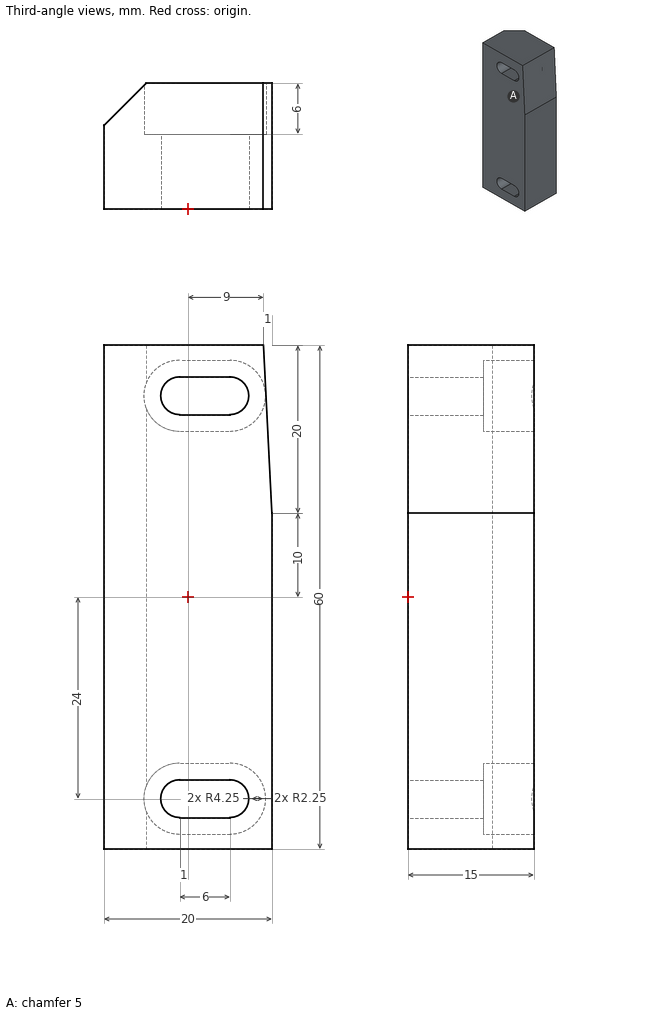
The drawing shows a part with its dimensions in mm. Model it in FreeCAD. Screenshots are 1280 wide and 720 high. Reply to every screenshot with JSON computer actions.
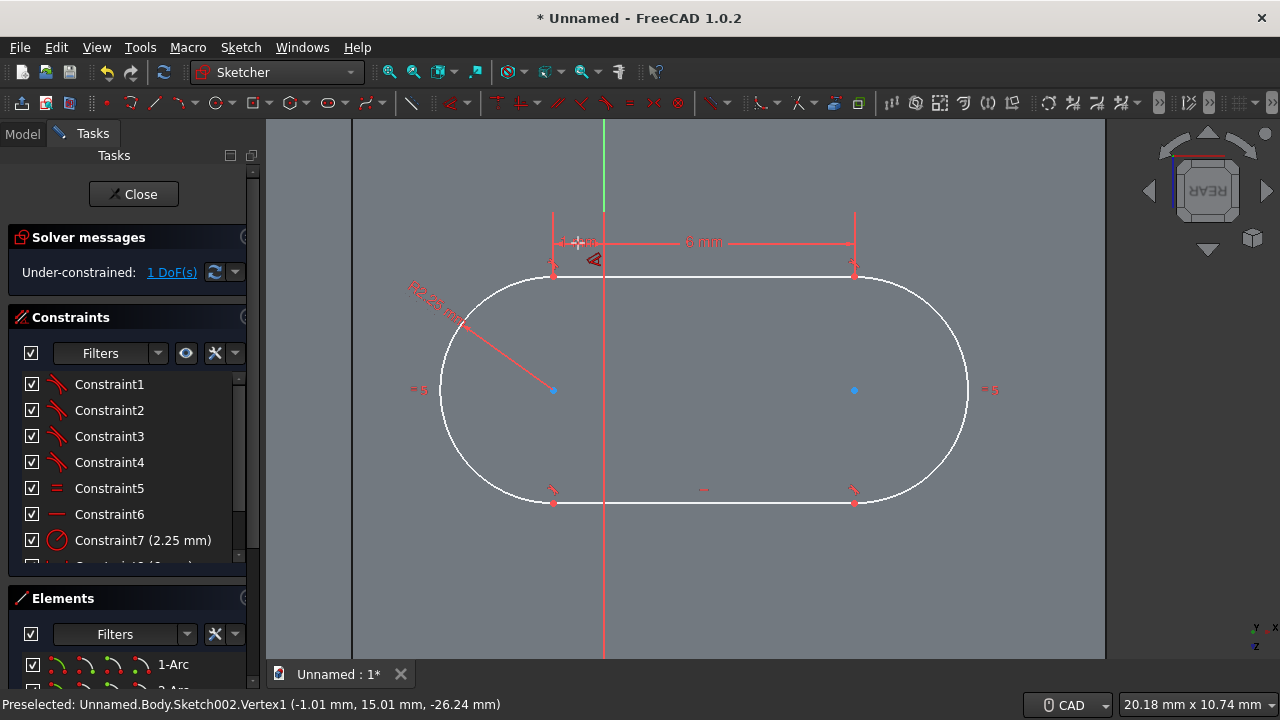
{"action": "left_click", "coordinate": [553, 390]}
{"action": "left_click", "coordinate": [519, 455]}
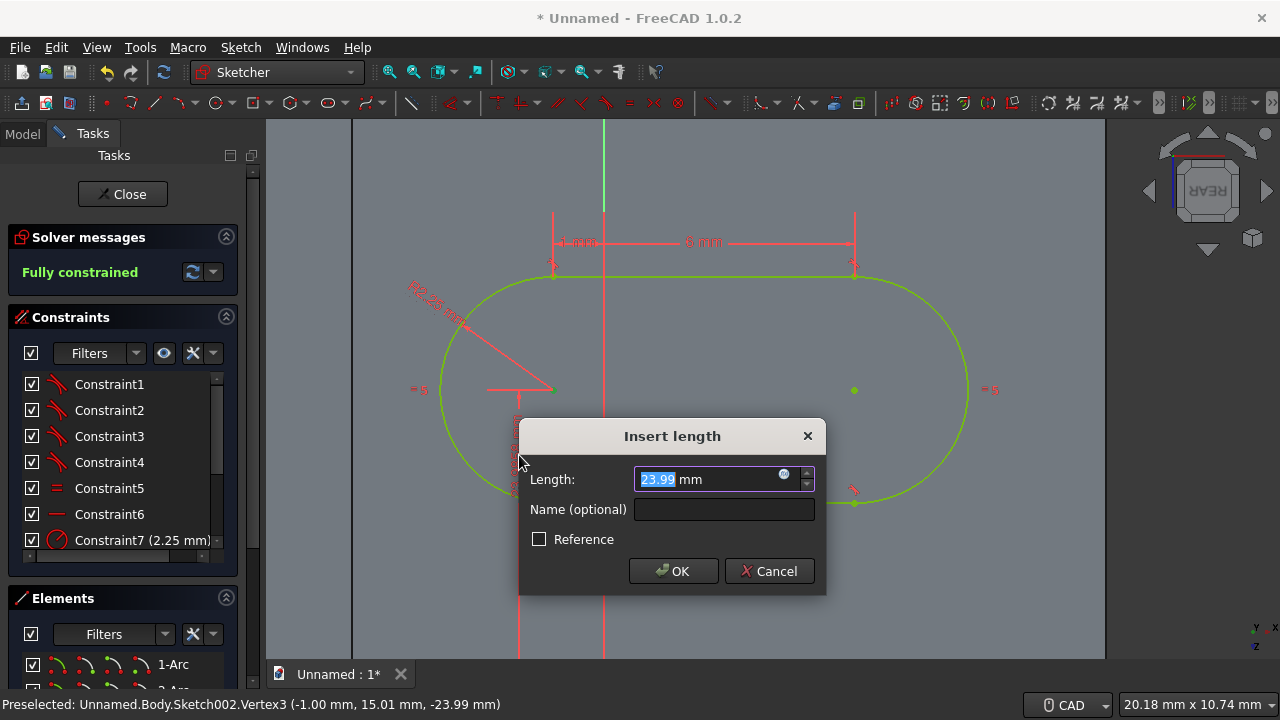
{"action": "type", "text": "24"}
{"action": "key", "text": "Return"}
{"action": "key", "text": "Escape"}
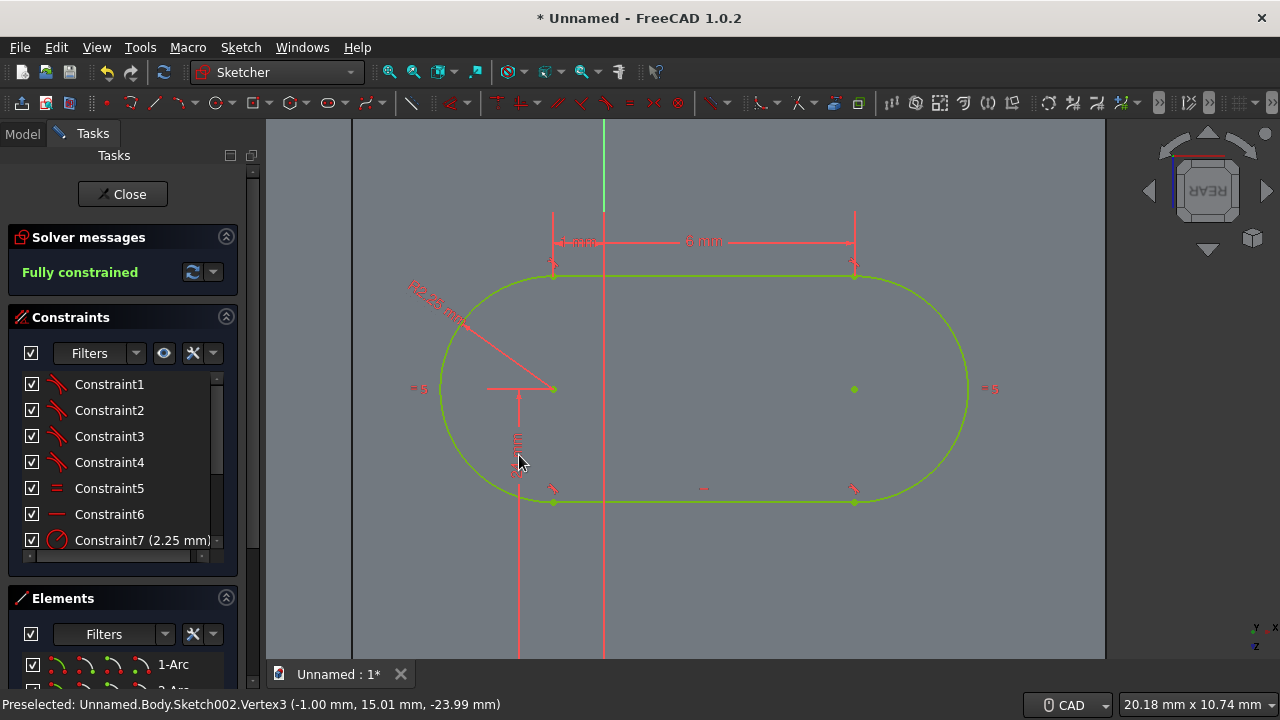
{"action": "left_click", "coordinate": [123, 194]}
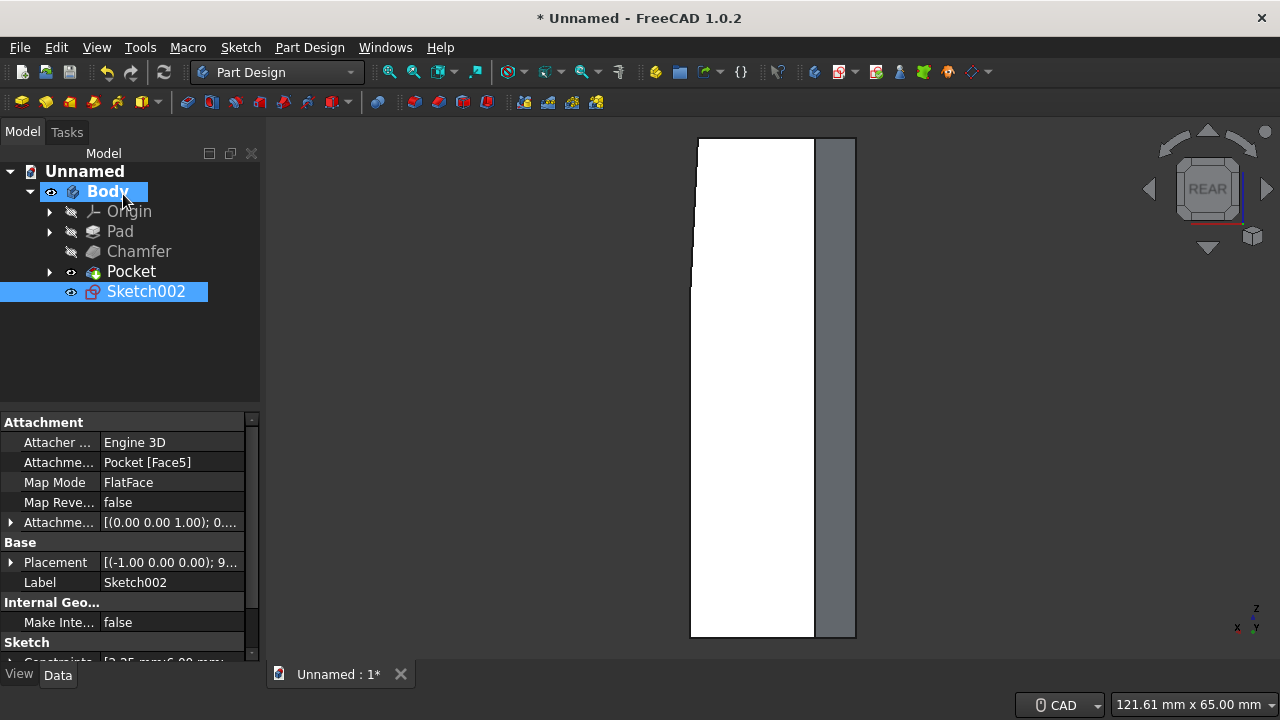
{"action": "left_click", "coordinate": [188, 102]}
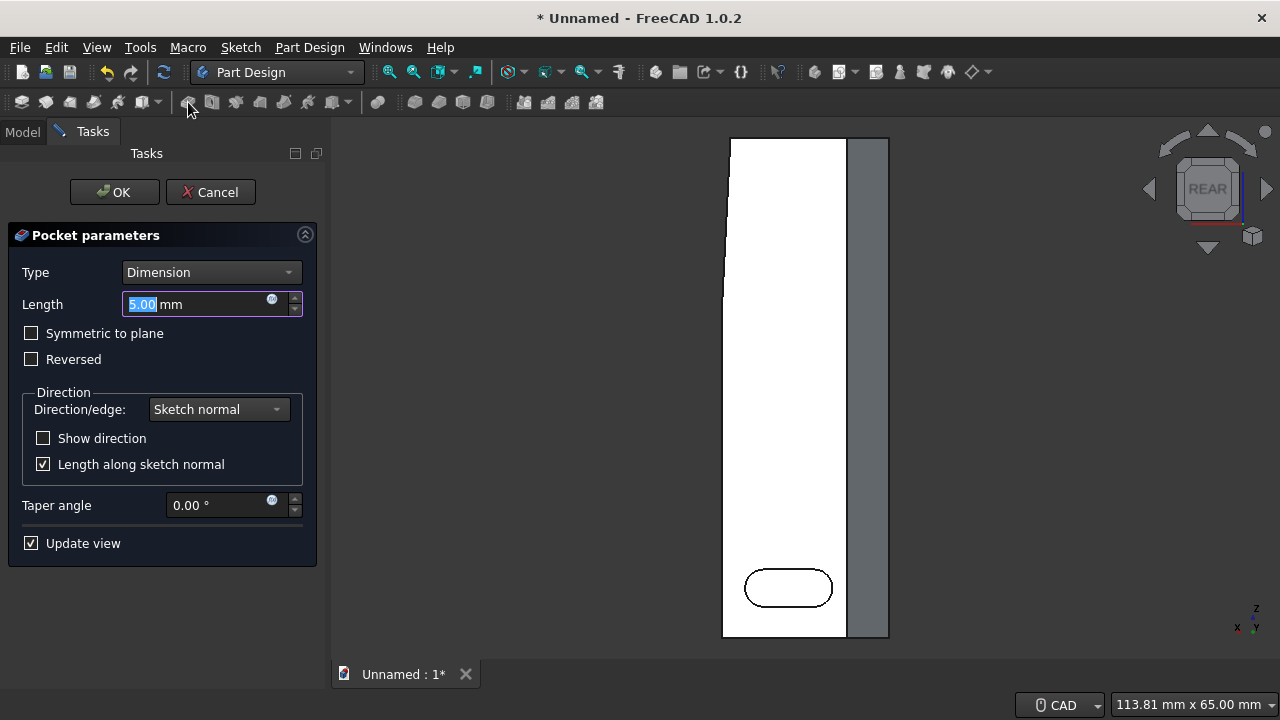
{"action": "left_click", "coordinate": [212, 272]}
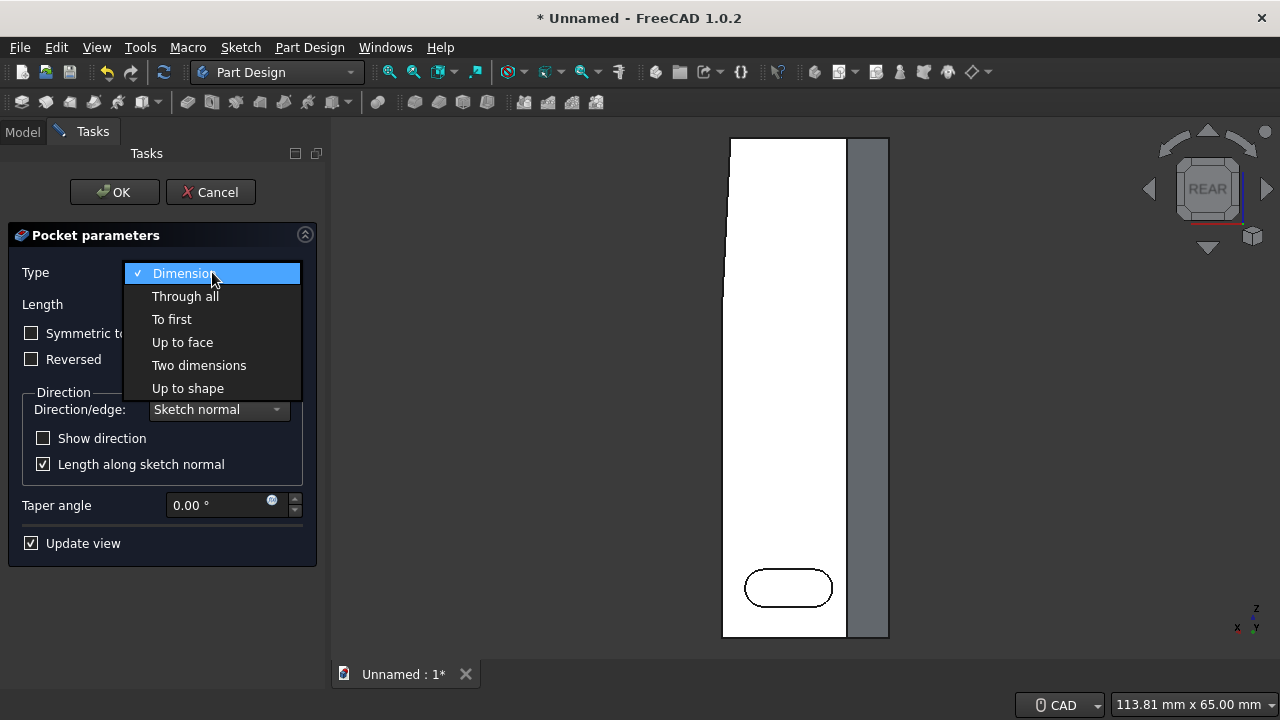
{"action": "left_click", "coordinate": [212, 296]}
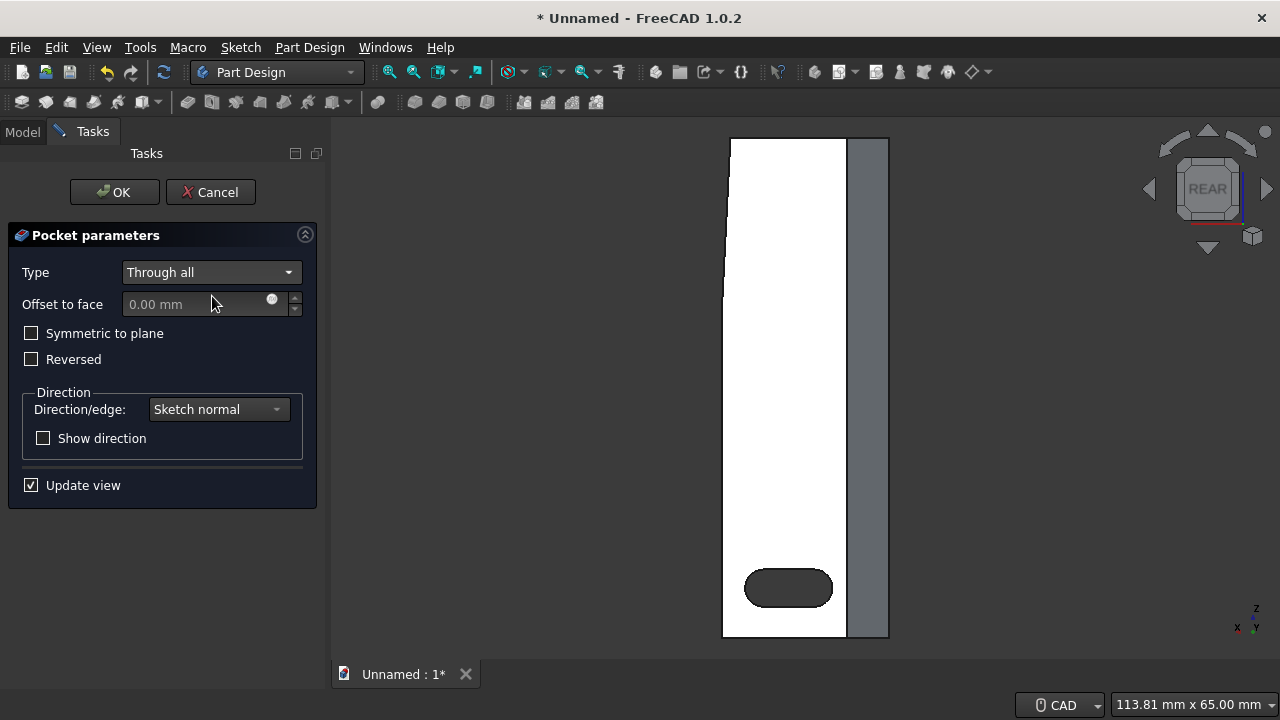
{"action": "left_click", "coordinate": [115, 192]}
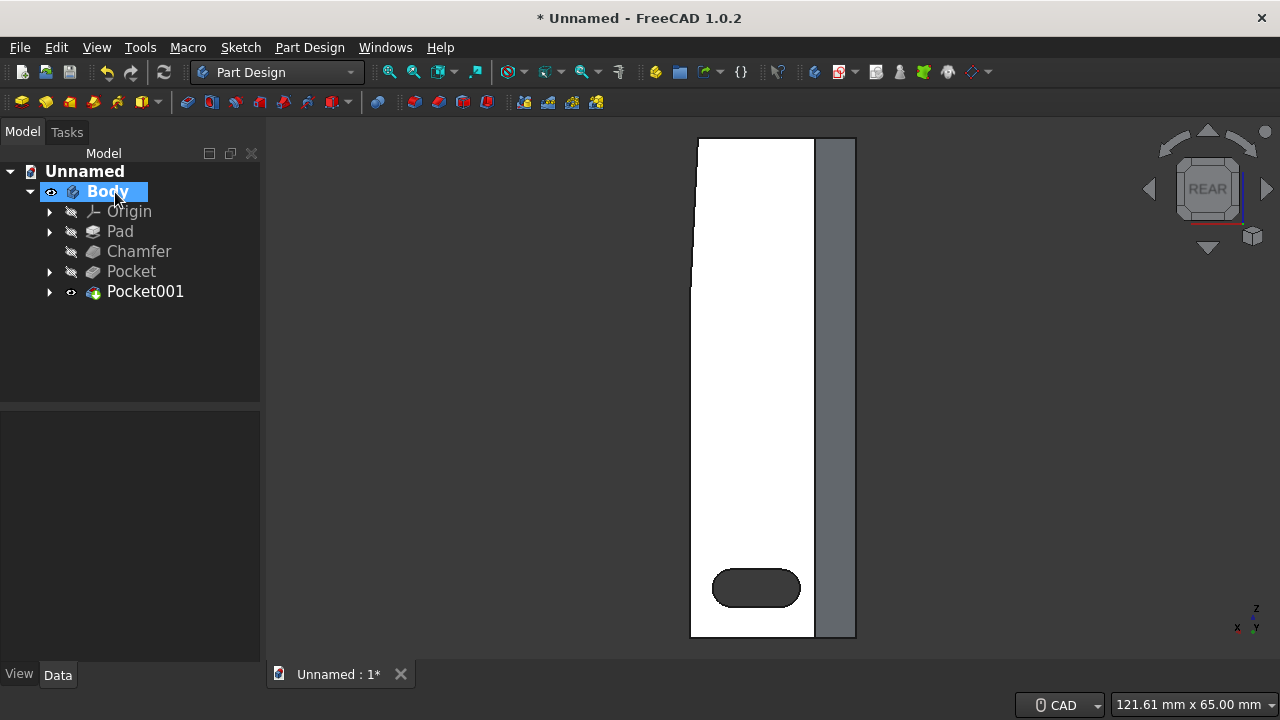
{"action": "left_click", "coordinate": [752, 316]}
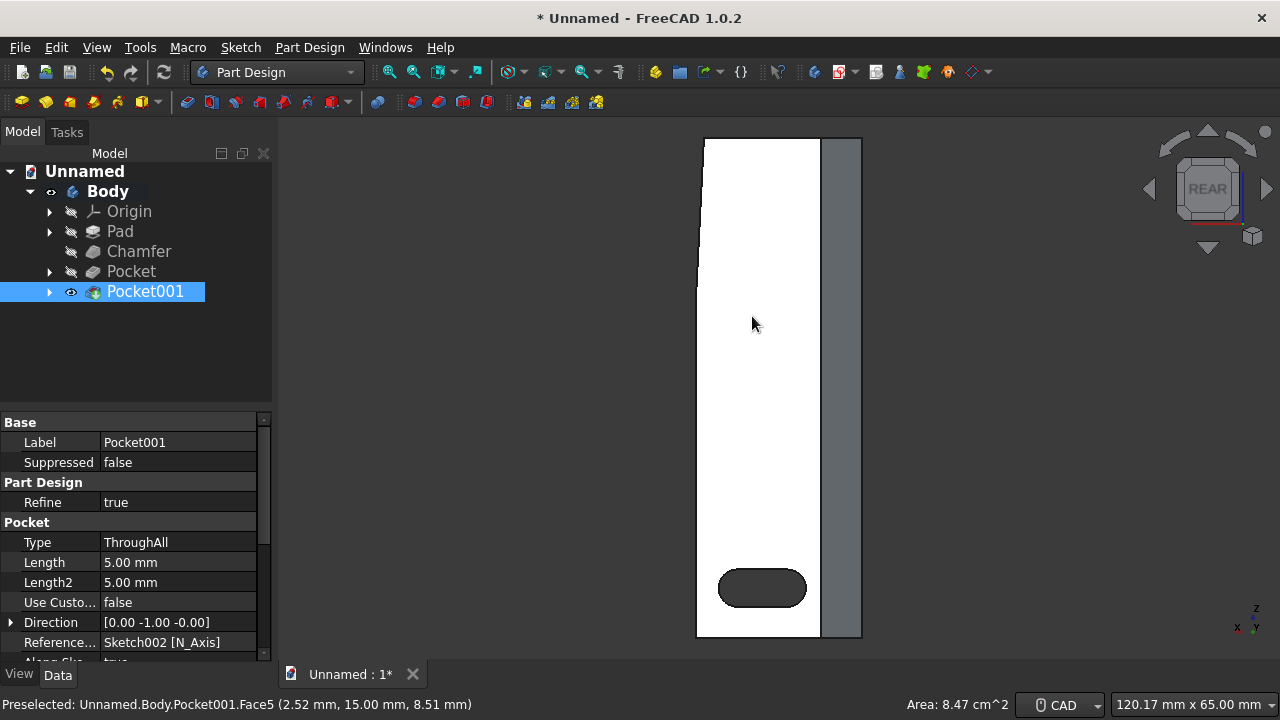
{"action": "left_click", "coordinate": [840, 72]}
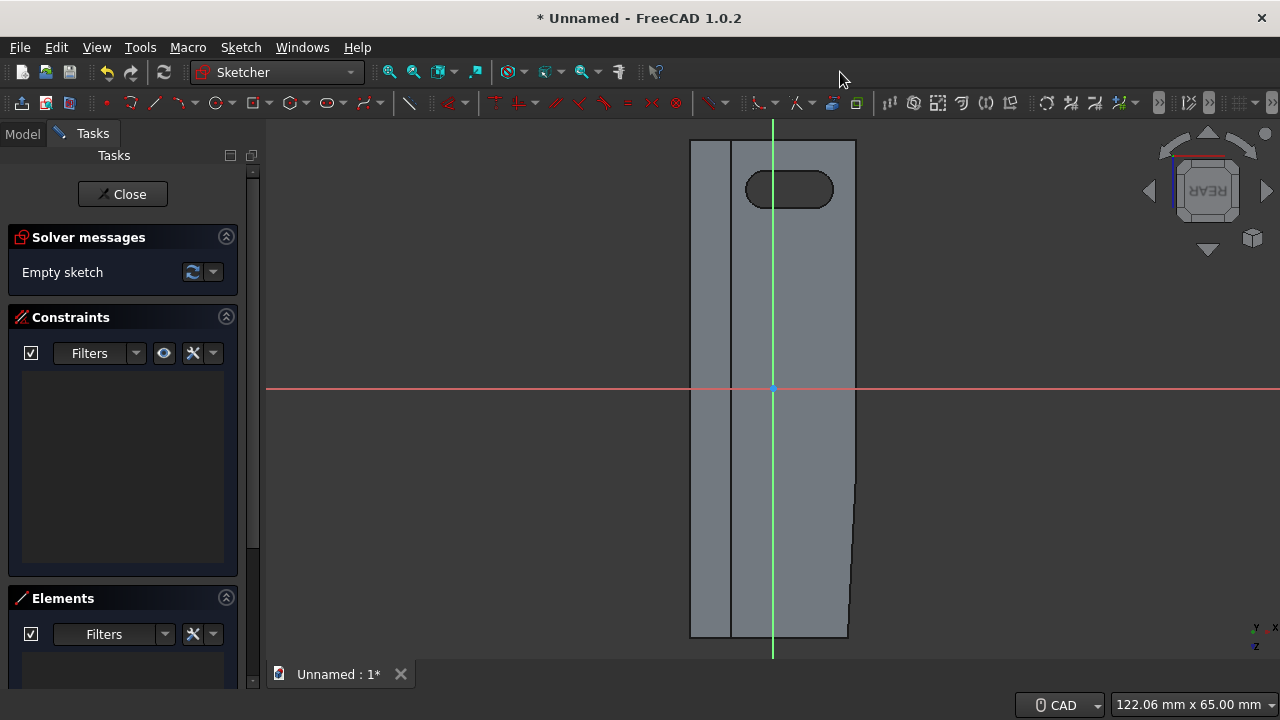
{"action": "scroll", "coordinate": [320, 631], "scroll_direction": "down", "scroll_amount": 1}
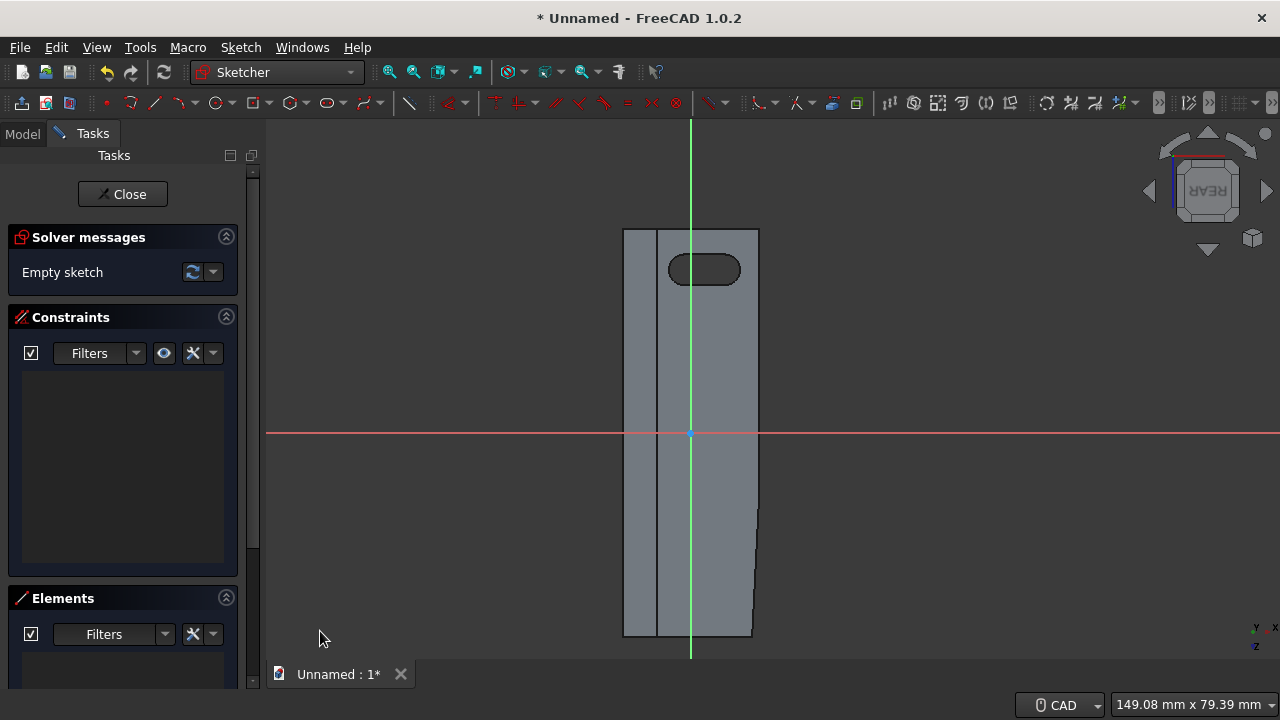
{"action": "scroll", "coordinate": [704, 274], "scroll_direction": "up", "scroll_amount": 3}